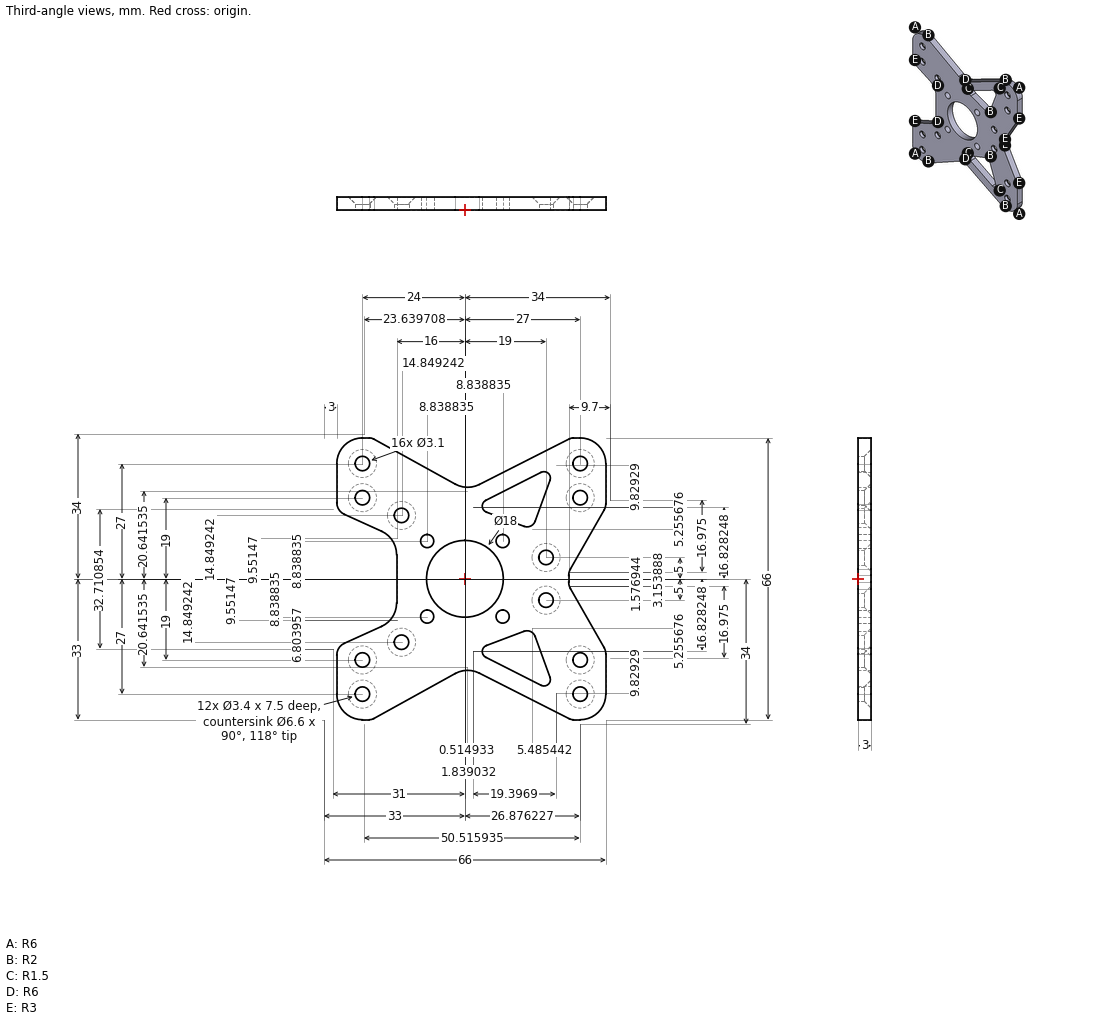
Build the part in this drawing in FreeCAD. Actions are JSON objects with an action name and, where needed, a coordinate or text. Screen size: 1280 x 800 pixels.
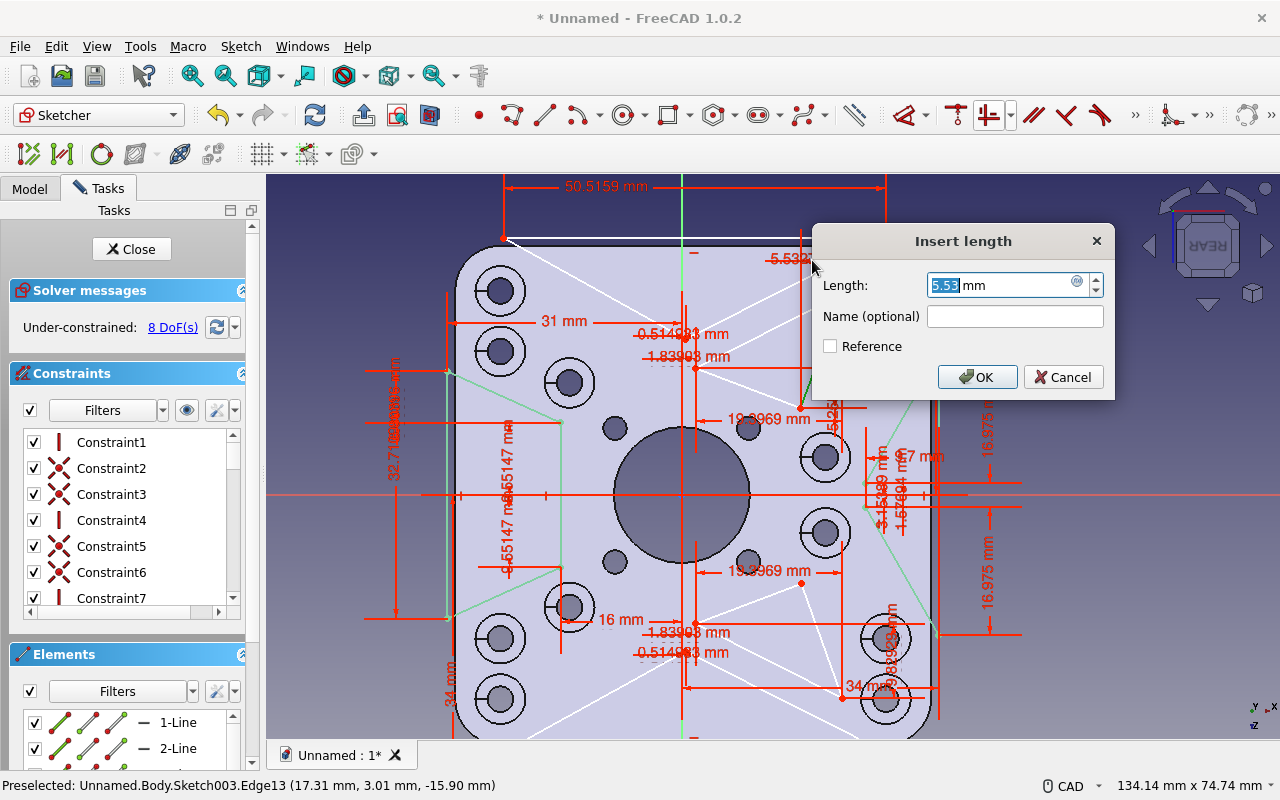
{"action": "type", "text": "5.485442"}
{"action": "key", "text": "Return"}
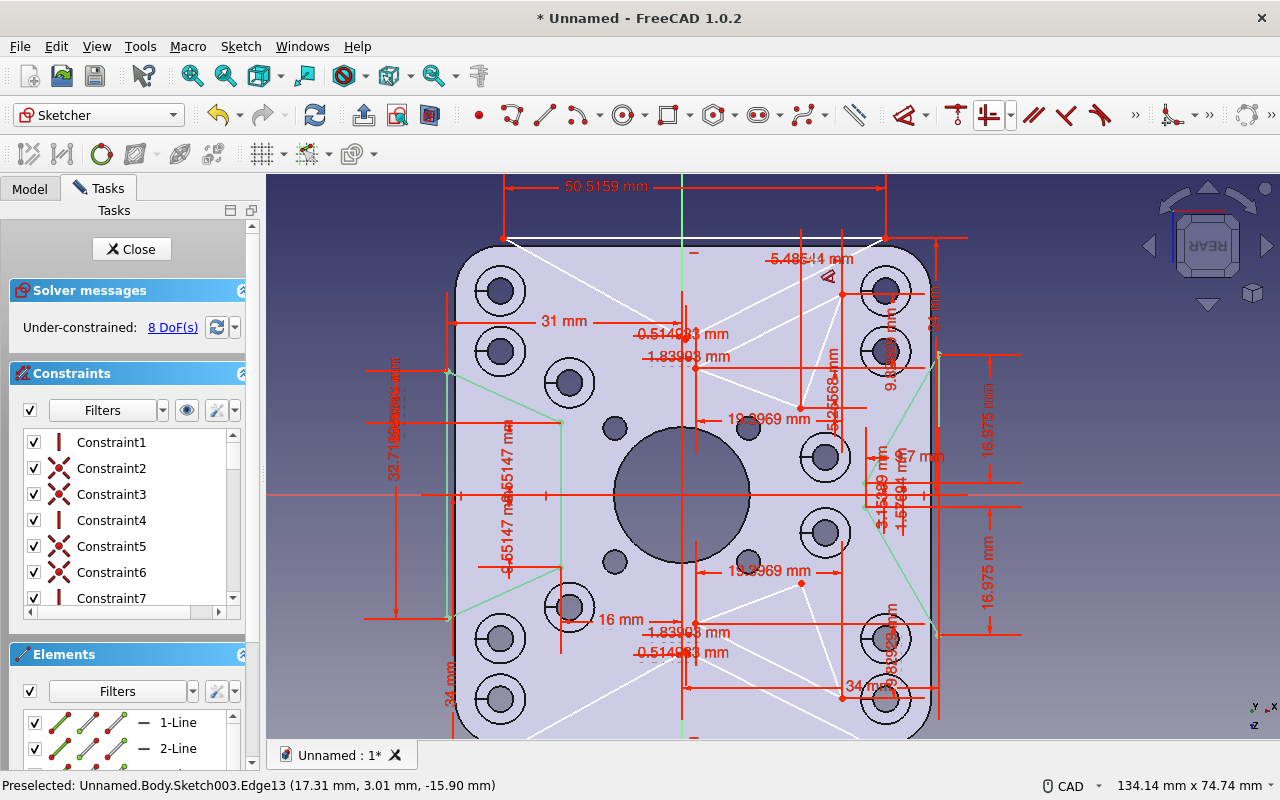
{"action": "left_click", "coordinate": [830, 664]}
{"action": "left_click", "coordinate": [822, 550]}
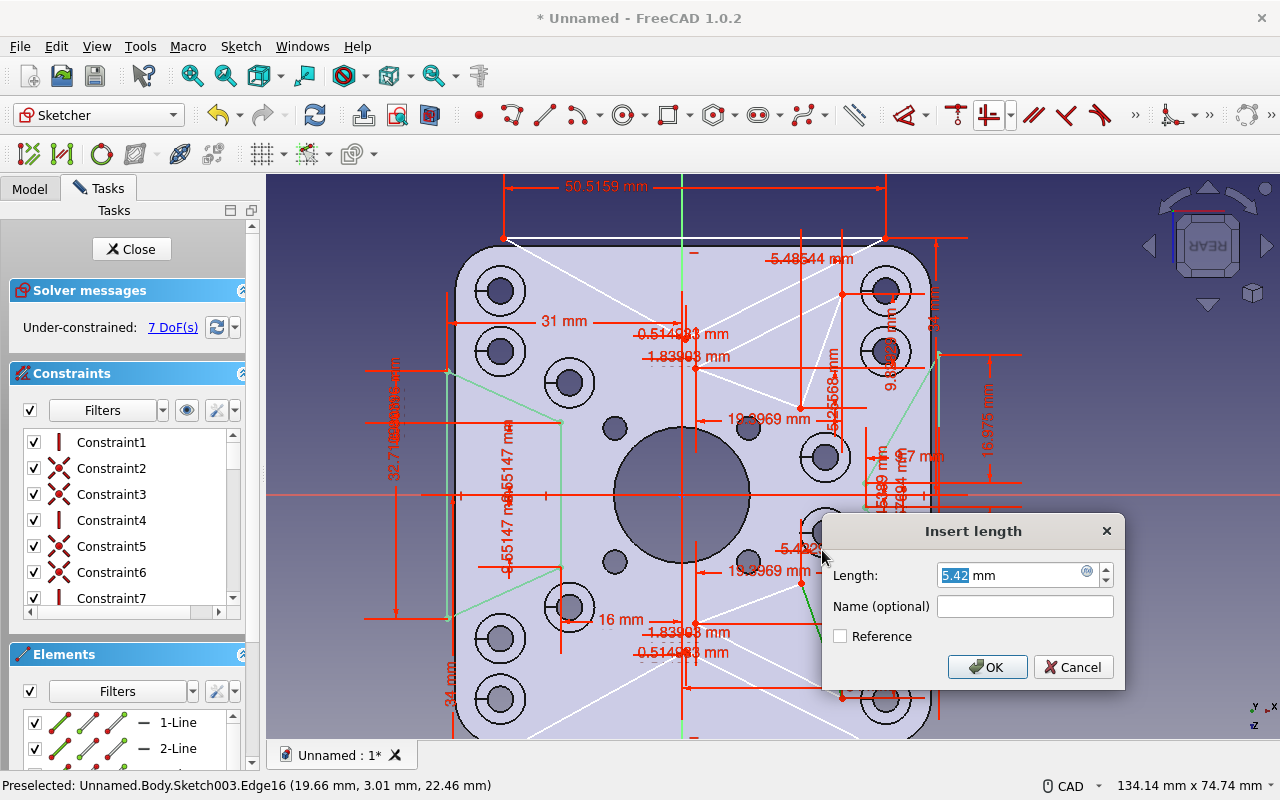
{"action": "type", "text": "5.485442"}
{"action": "key", "text": "Return"}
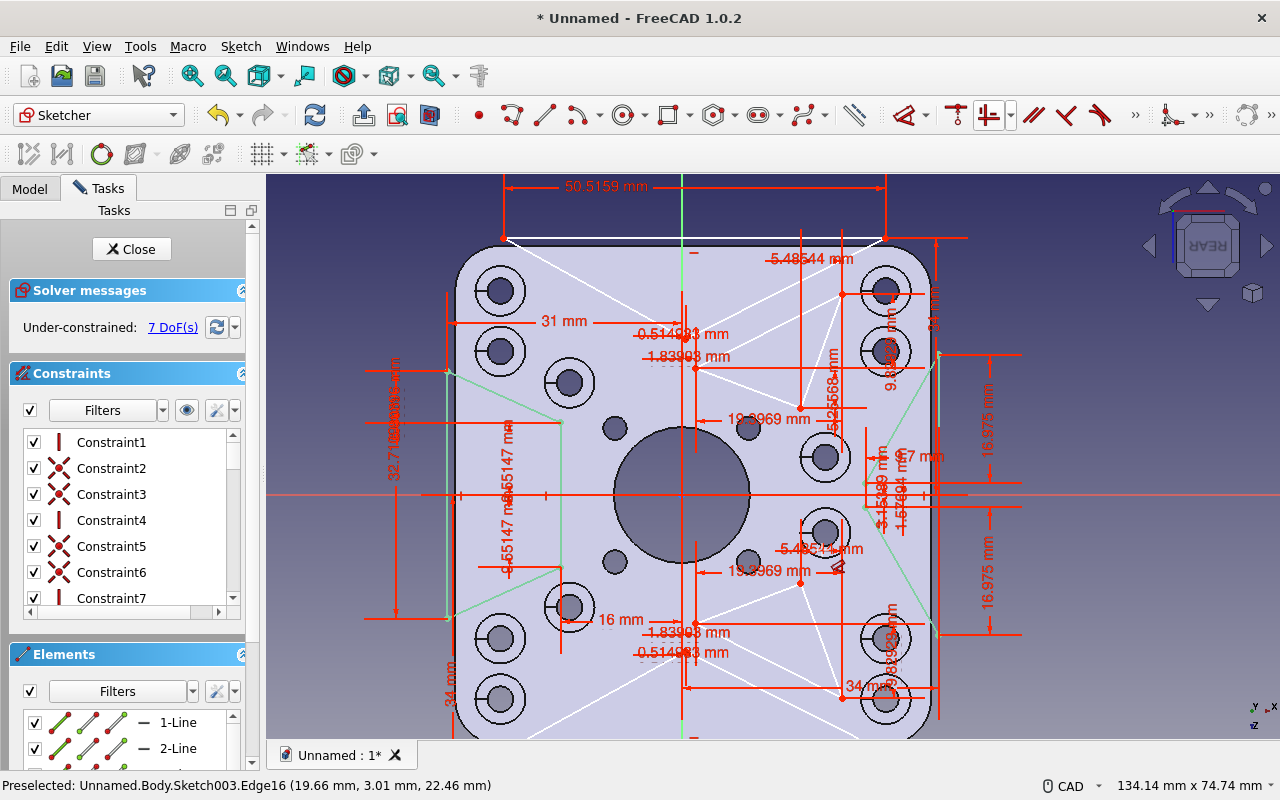
{"action": "left_click", "coordinate": [769, 596]}
{"action": "left_click", "coordinate": [835, 604]}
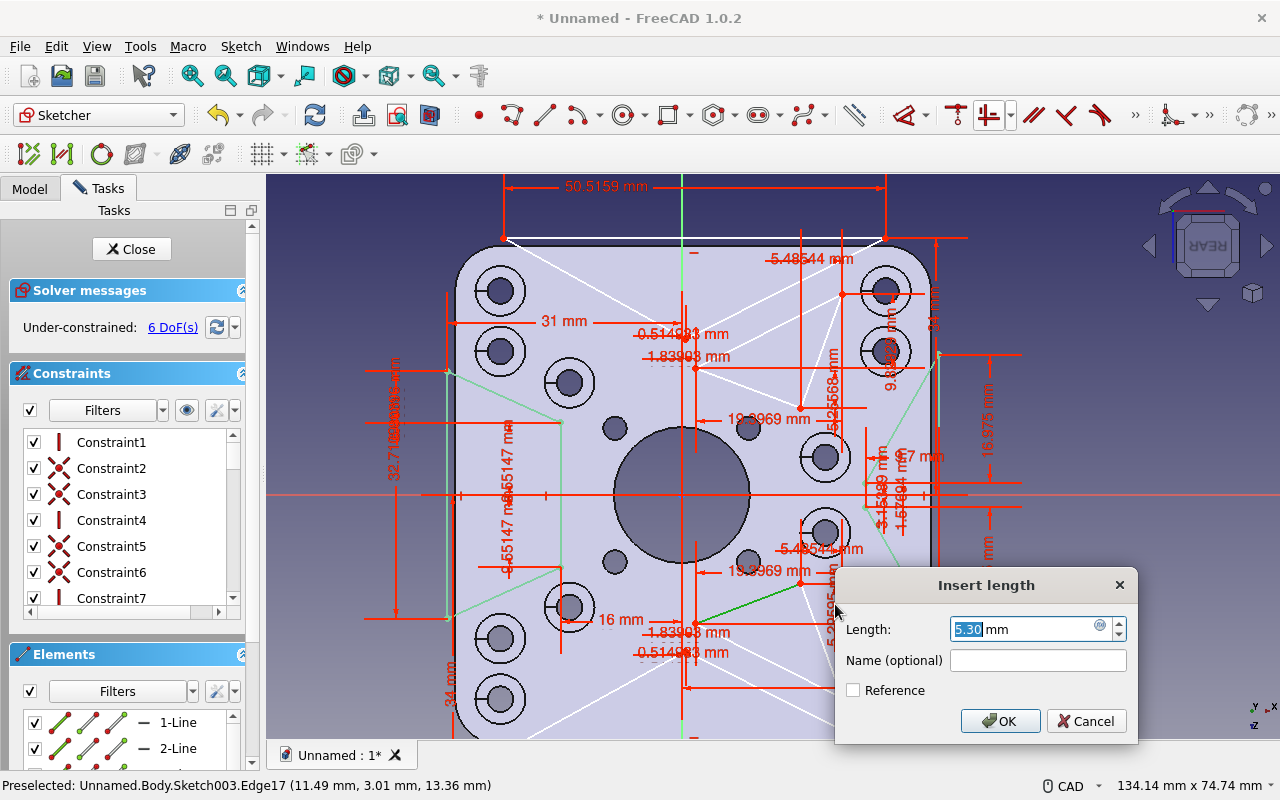
{"action": "type", "text": "5.255676"}
{"action": "key", "text": "Return"}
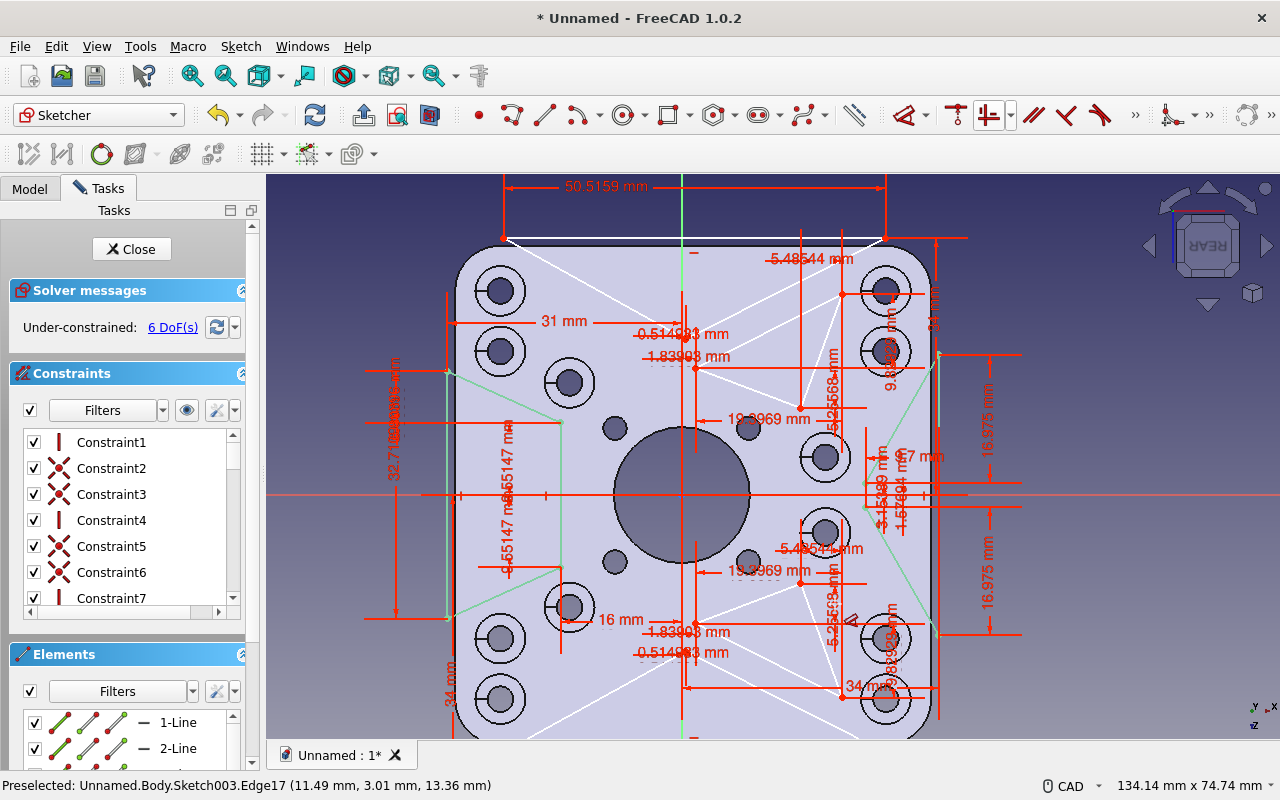
{"action": "left_click", "coordinate": [686, 339]}
{"action": "left_click", "coordinate": [648, 417]}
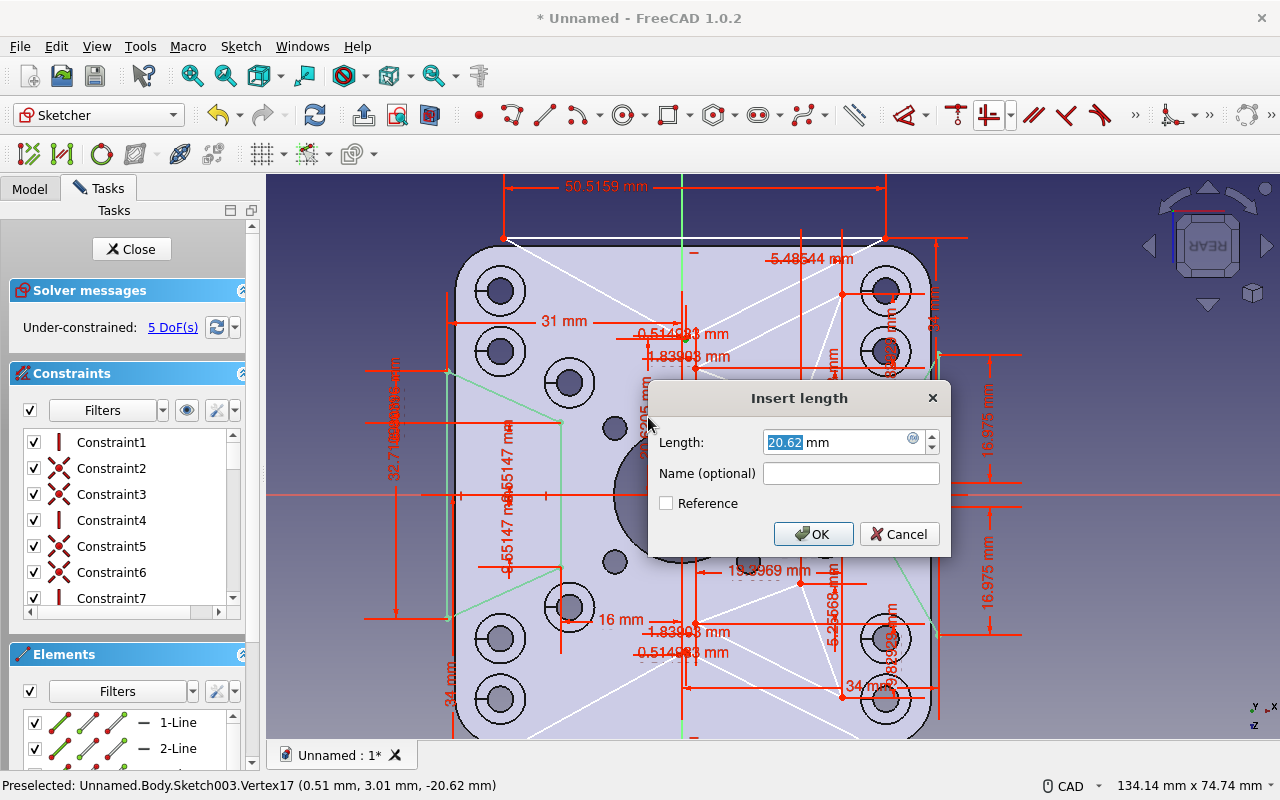
{"action": "type", "text": "20.641535"}
{"action": "key", "text": "Return"}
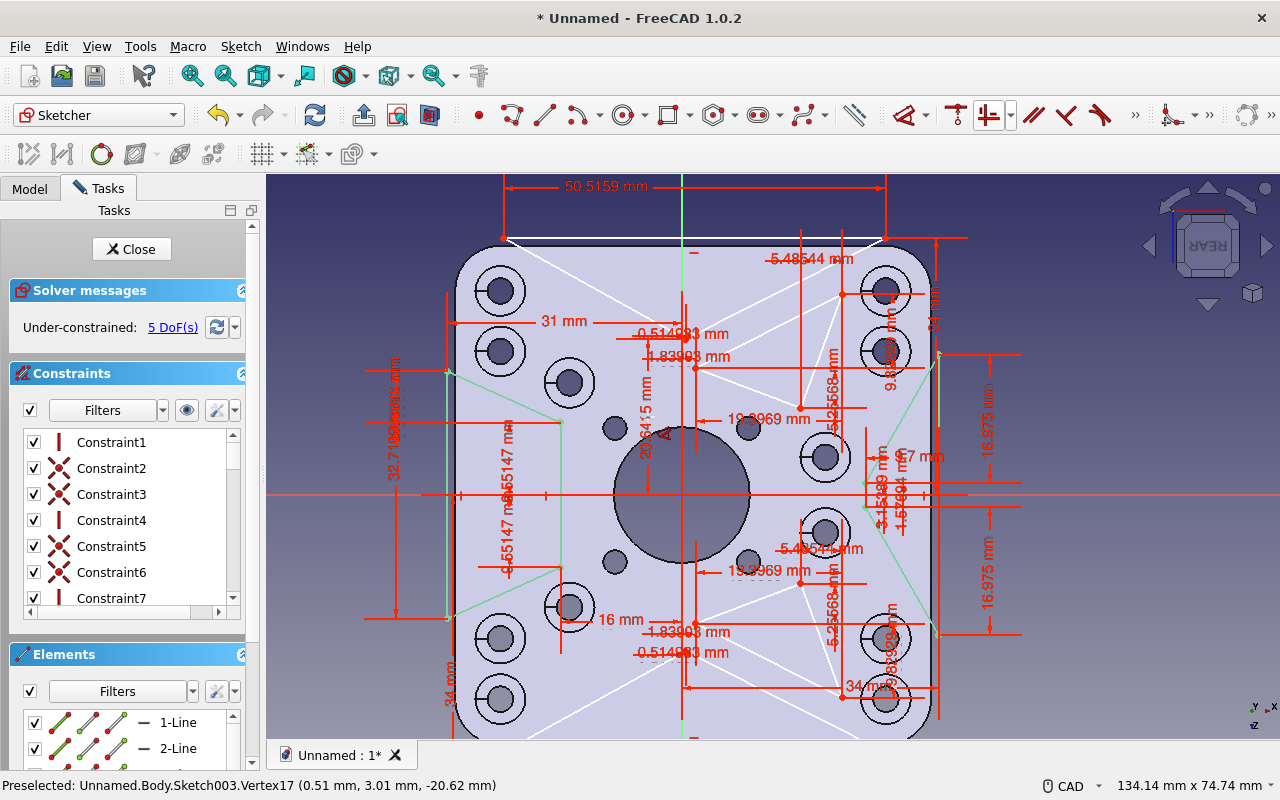
{"action": "left_click", "coordinate": [886, 238]}
{"action": "left_click", "coordinate": [784, 204]}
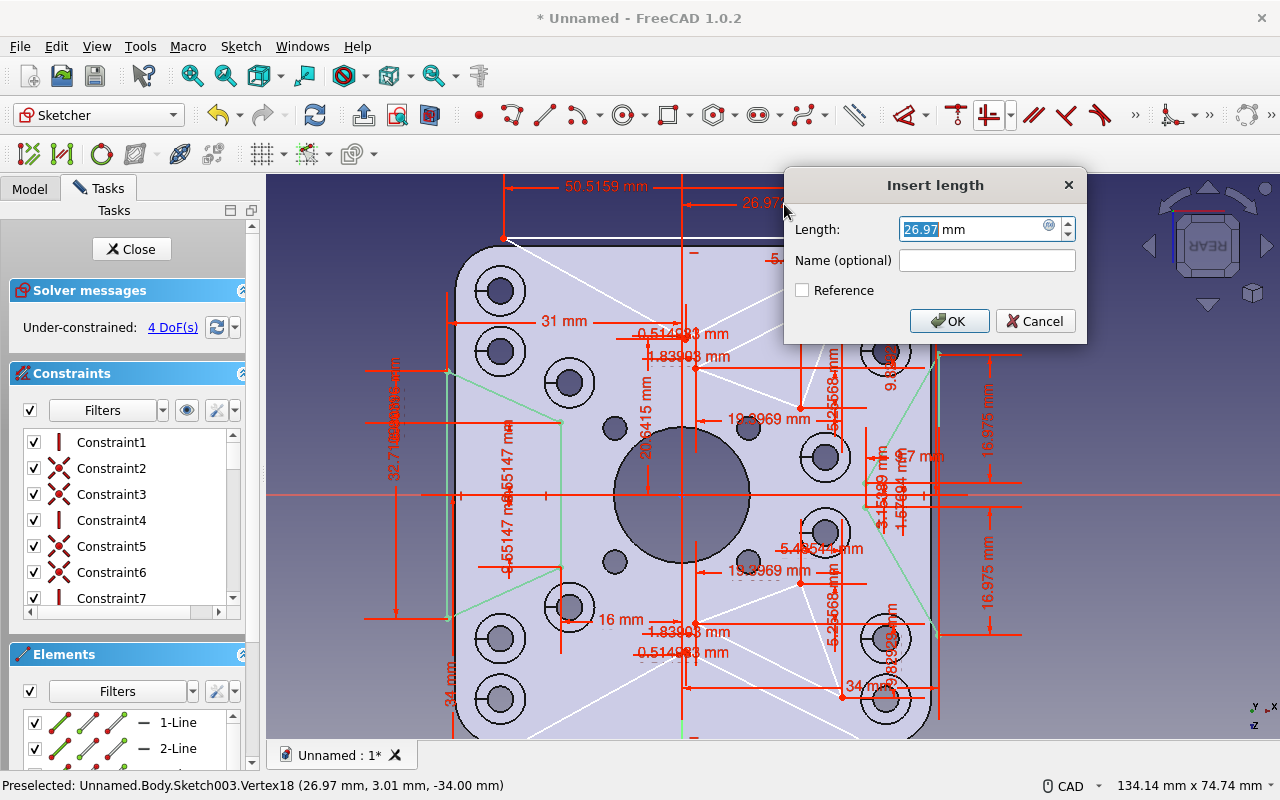
{"action": "type", "text": "26.876227"}
{"action": "key", "text": "Return"}